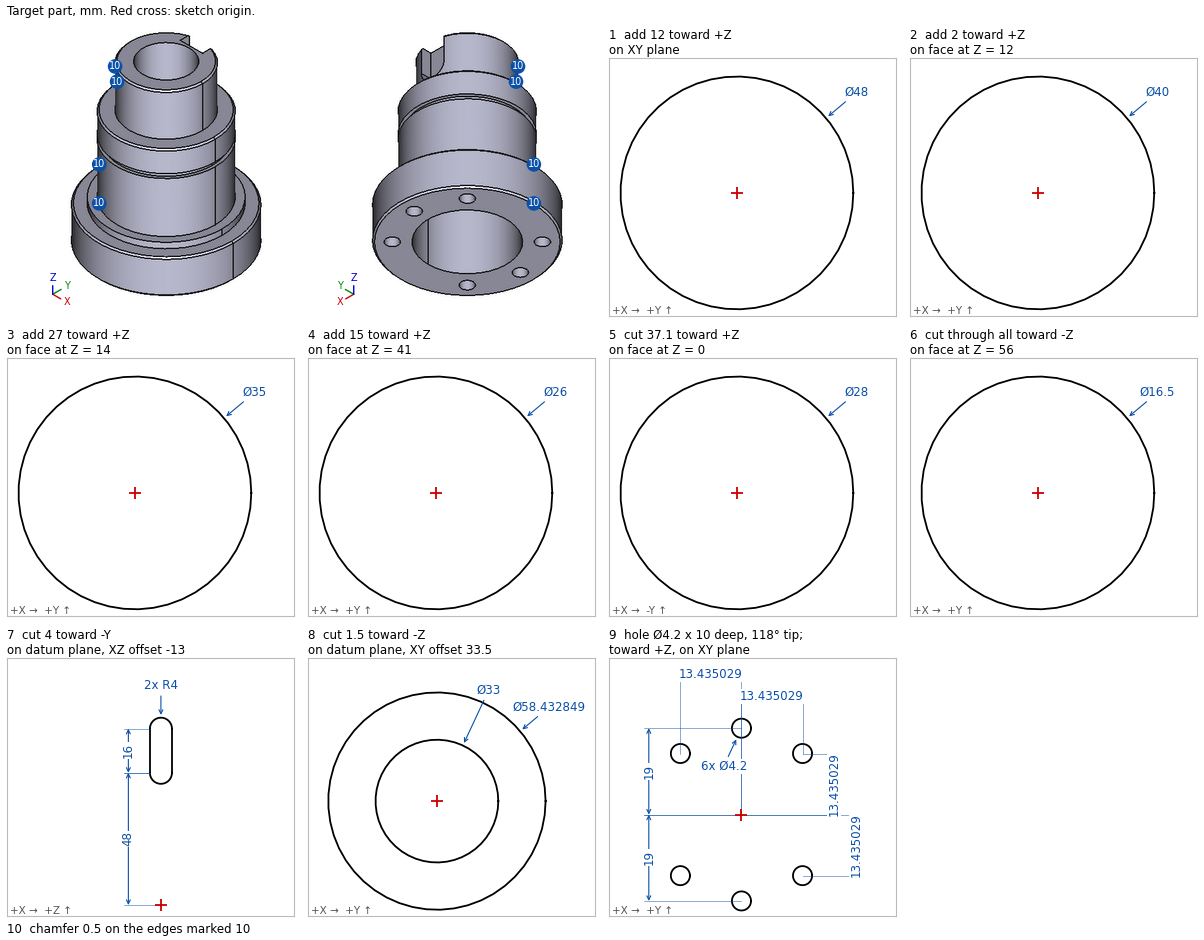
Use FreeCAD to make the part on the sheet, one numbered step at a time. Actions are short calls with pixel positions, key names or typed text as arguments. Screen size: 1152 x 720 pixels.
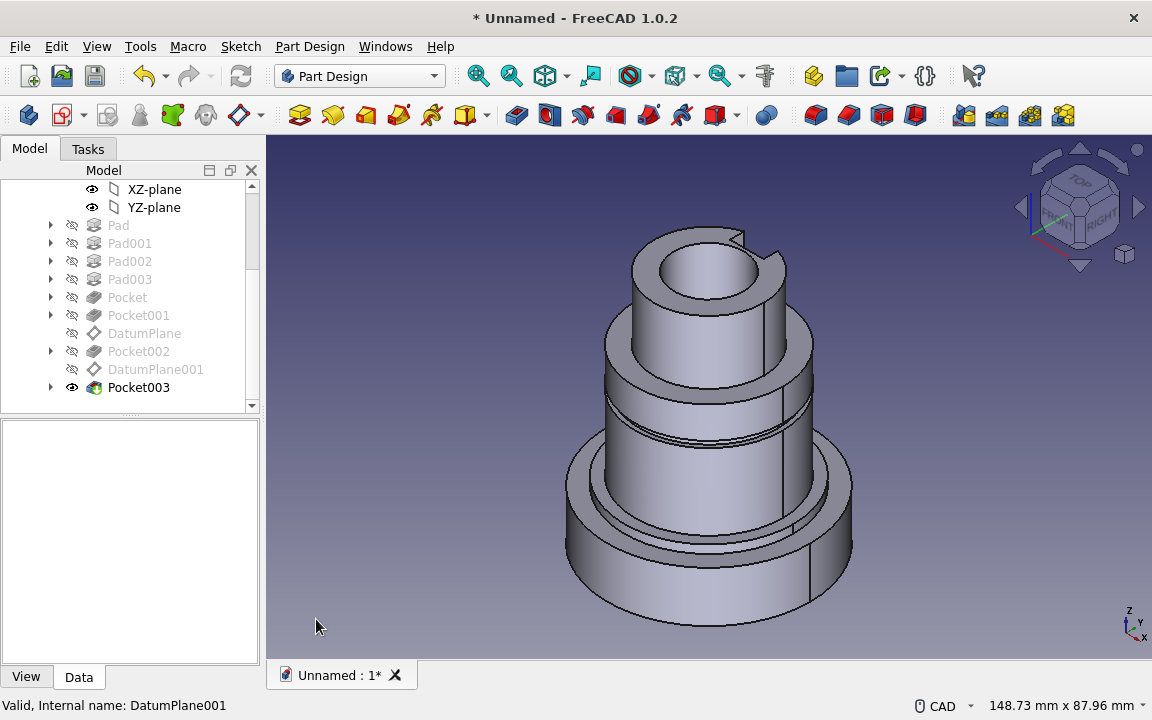
click(62, 116)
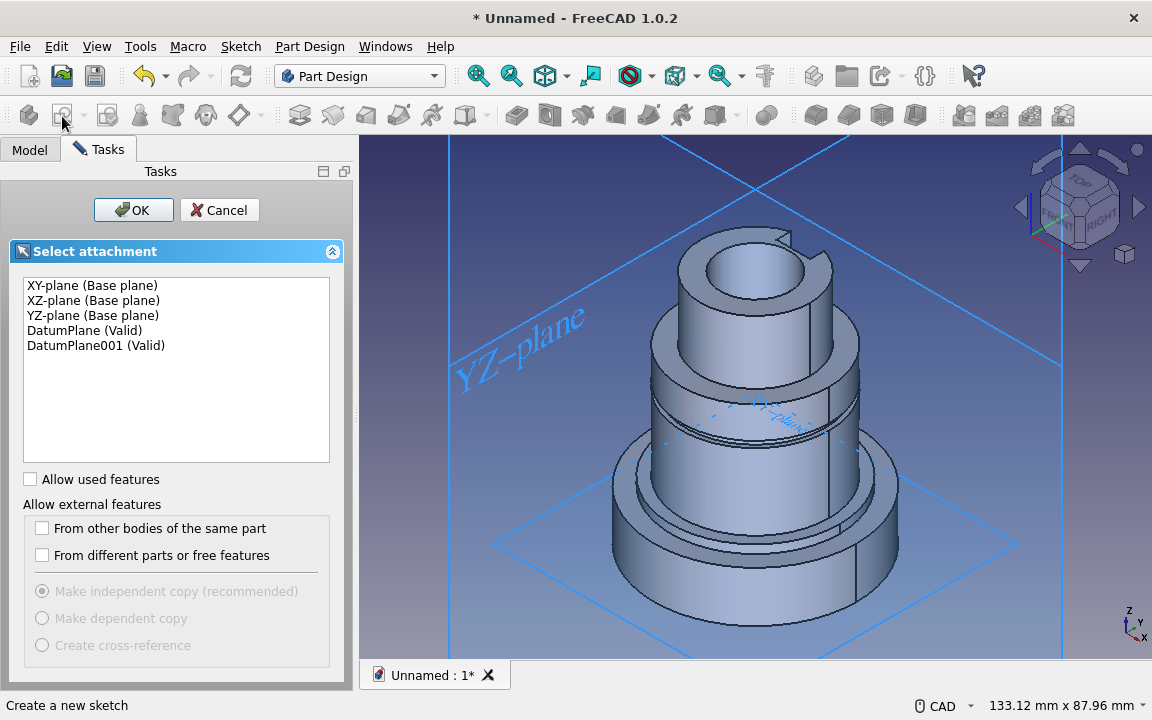
click(84, 286)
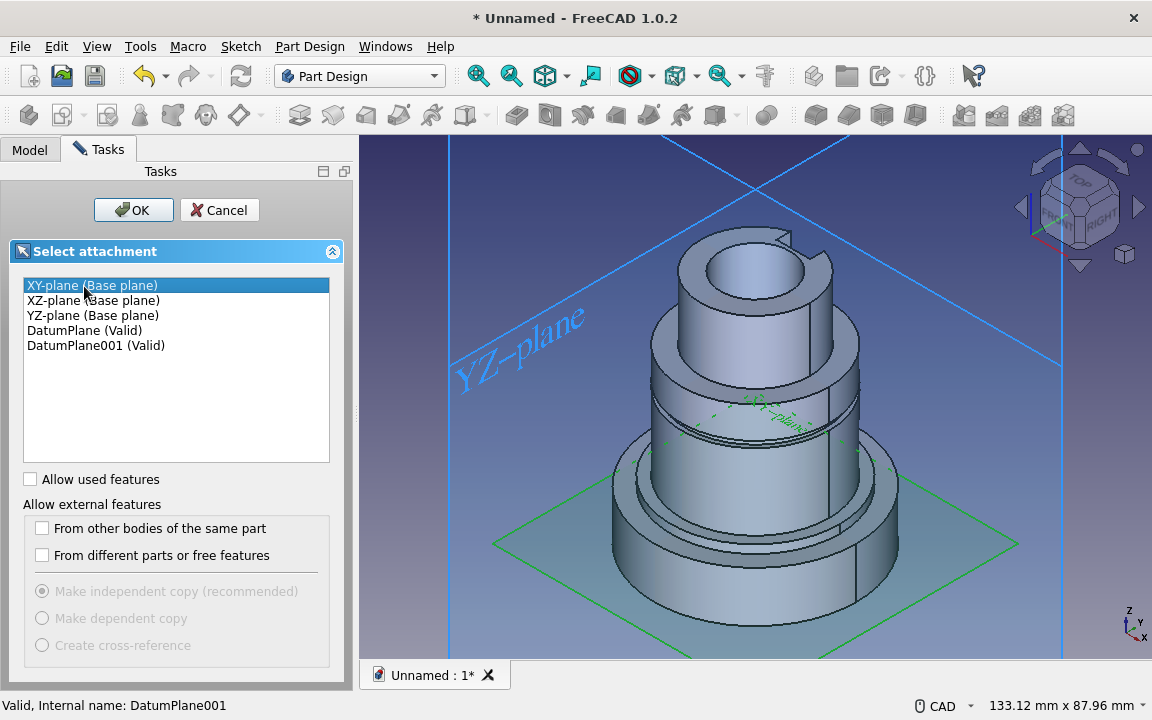
click(134, 210)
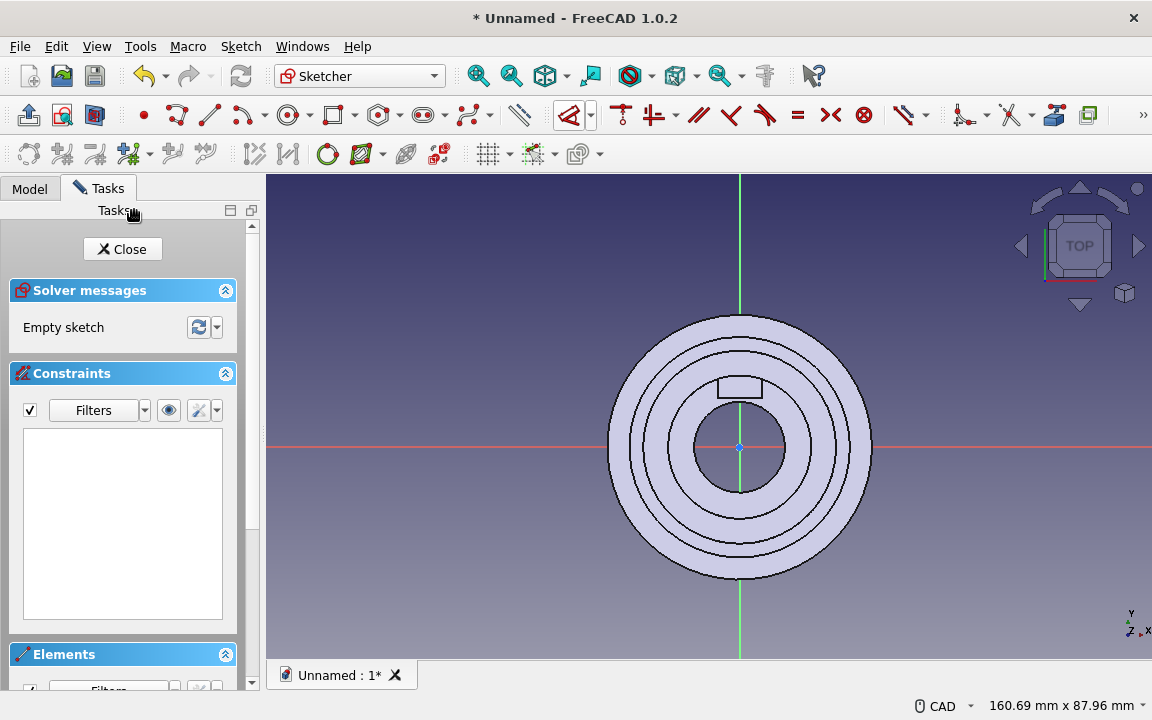
key(q)
key(s)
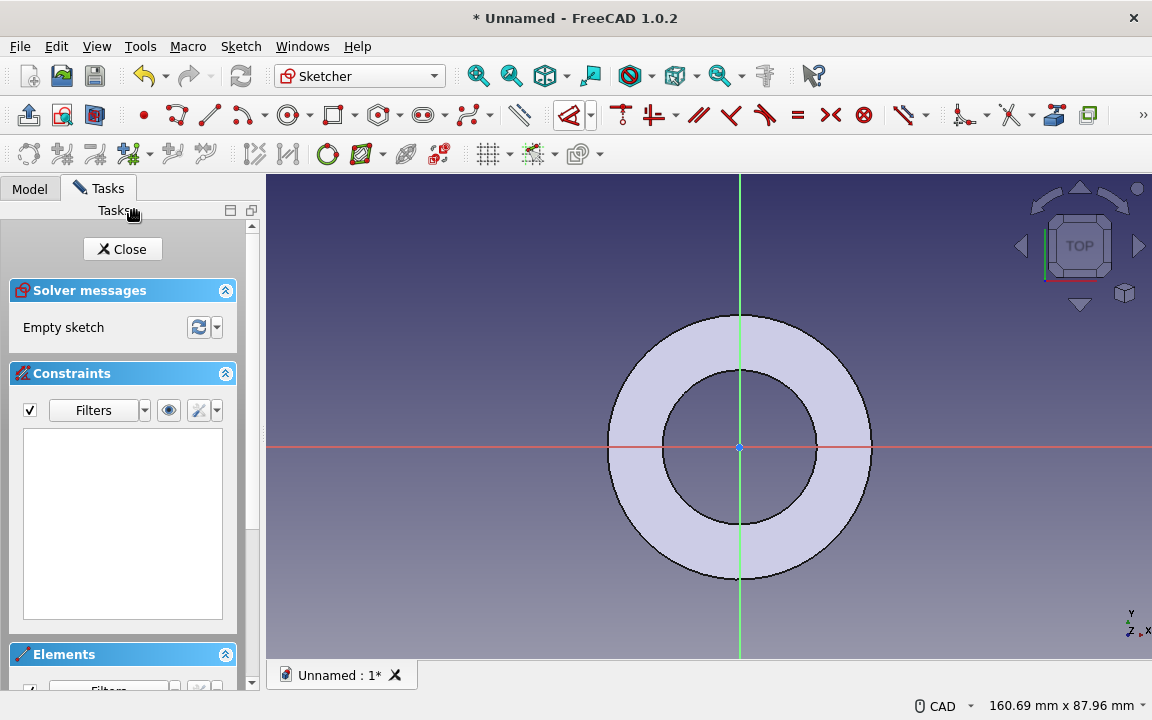
key(g)
key(c)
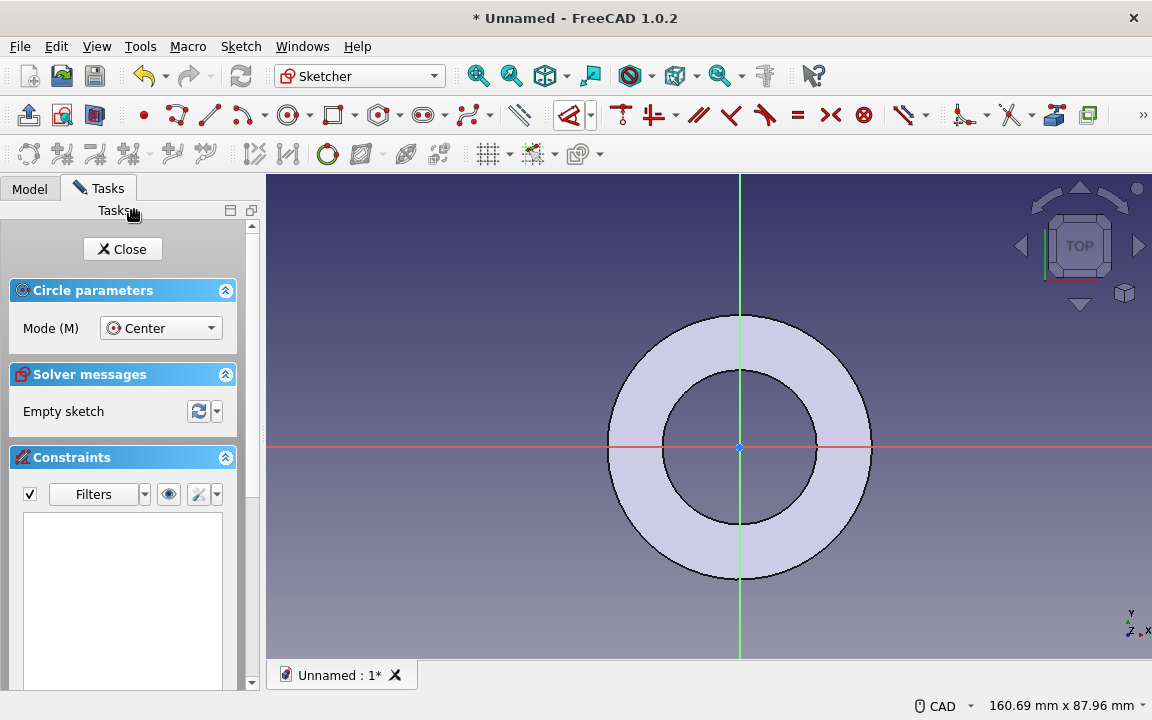
scroll(740, 343, up, 4)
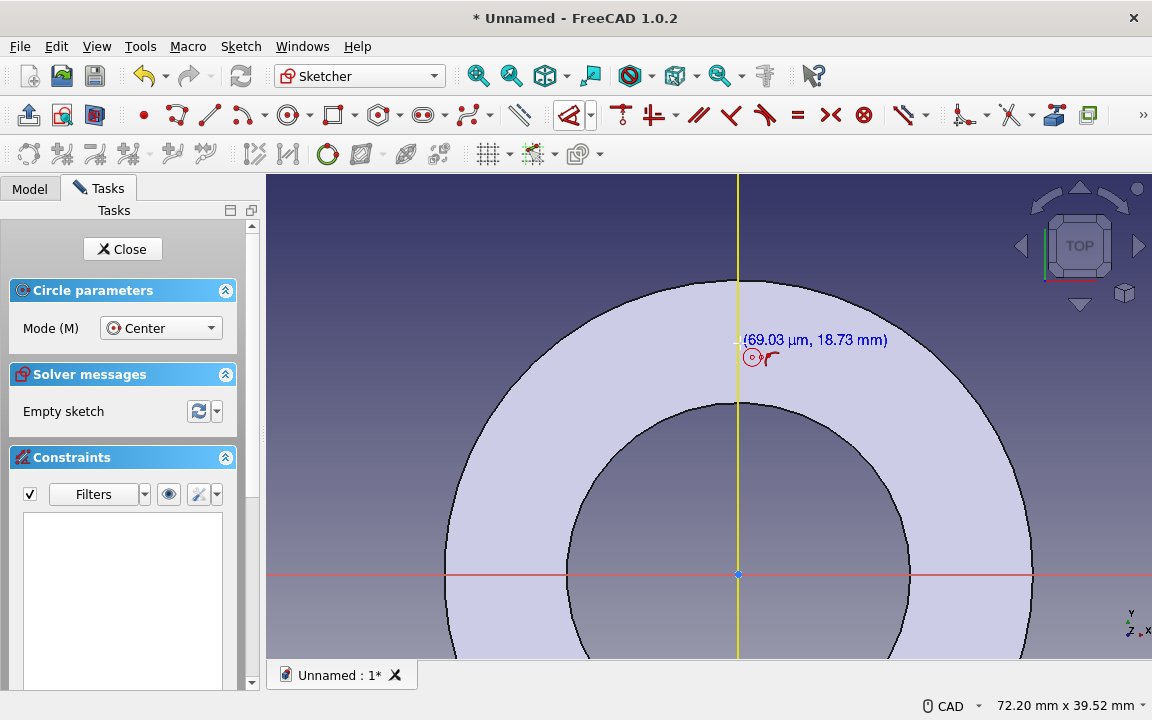
click(738, 341)
click(757, 323)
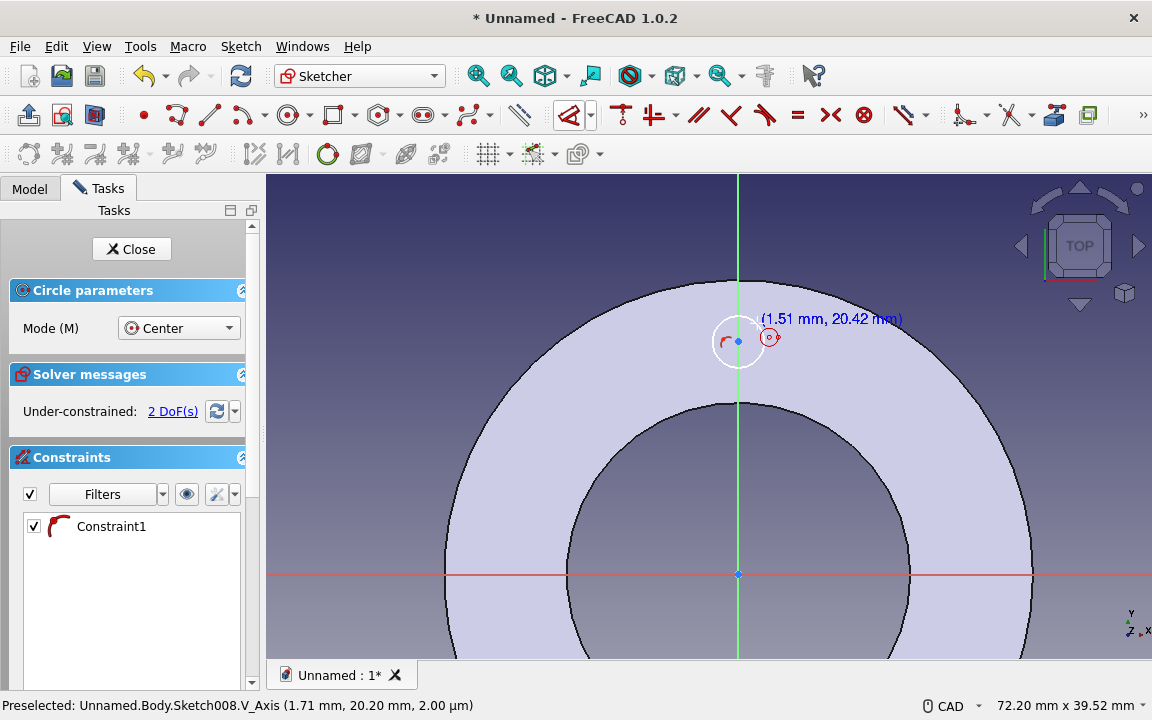
click(903, 410)
click(922, 392)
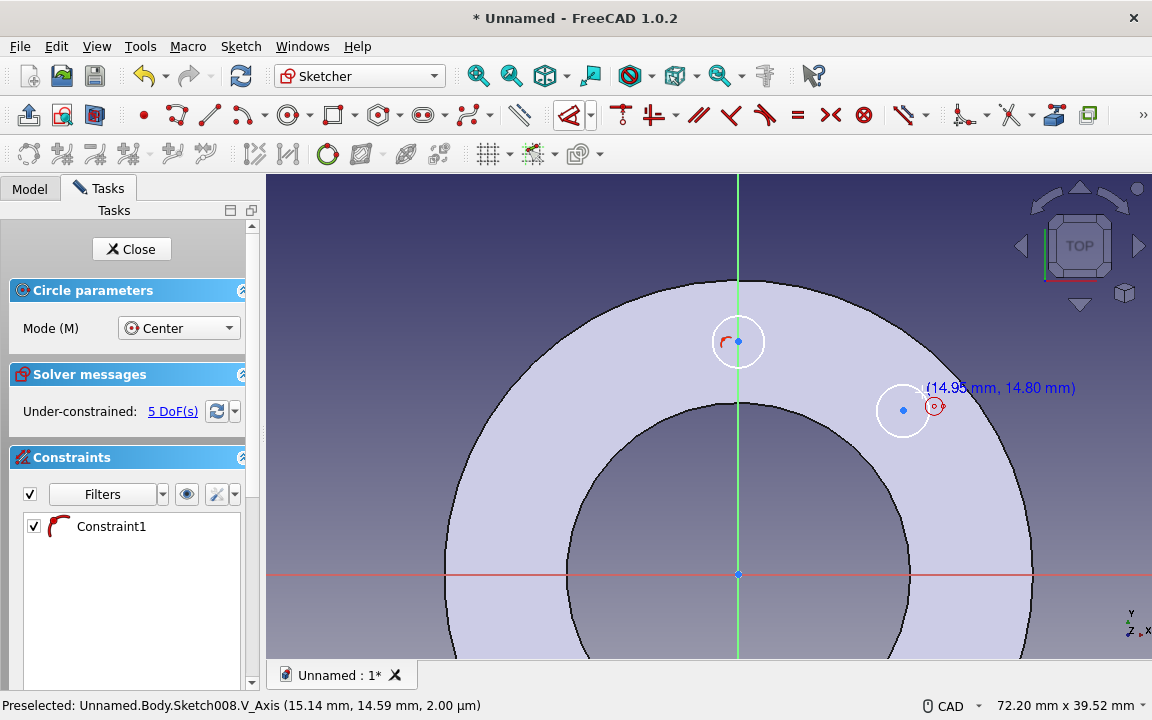
click(574, 410)
click(592, 392)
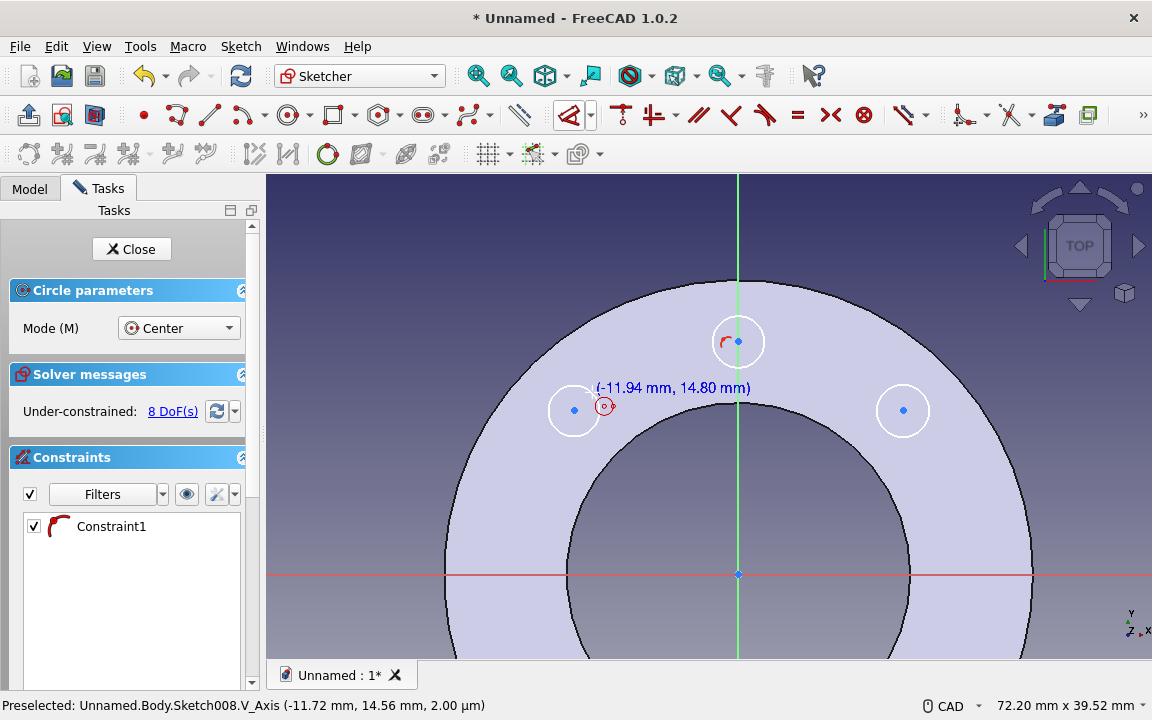
scroll(521, 224, down, 3)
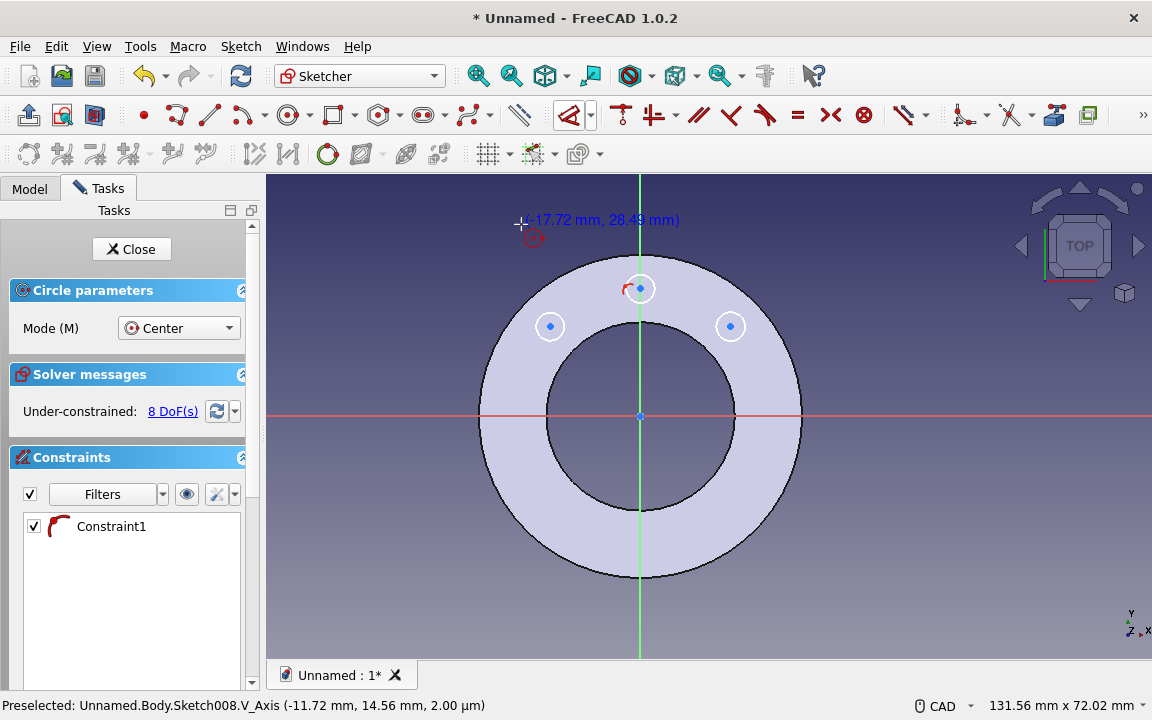
scroll(731, 507, up, 3)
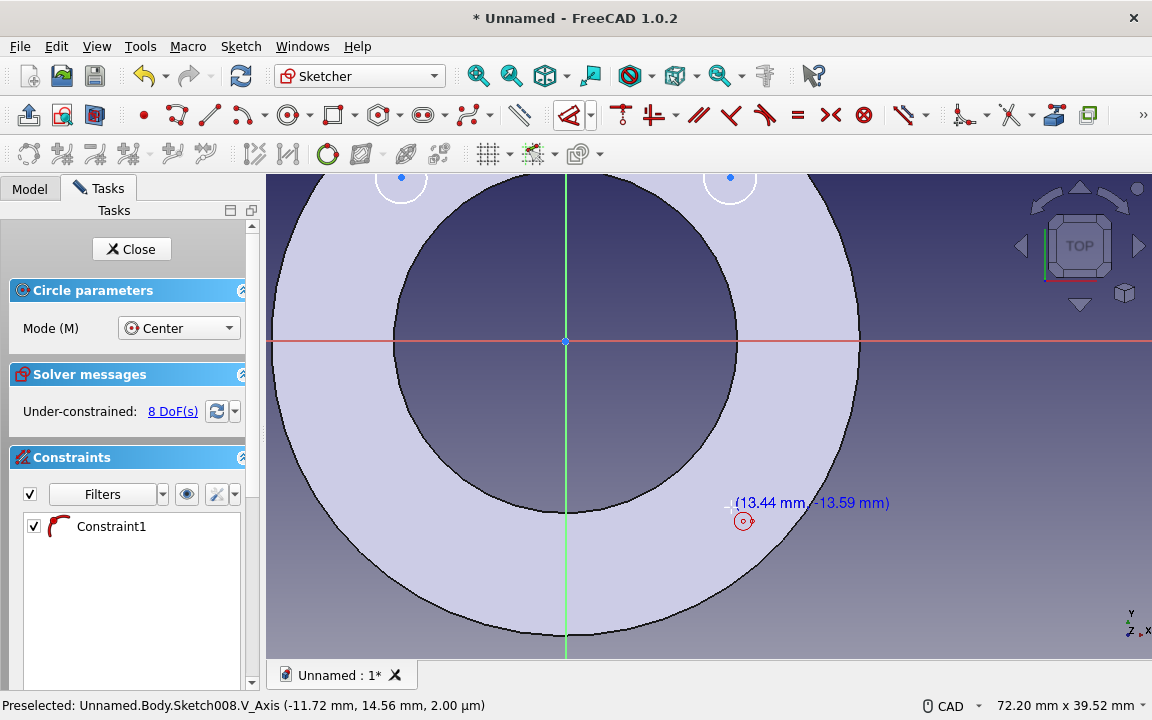
click(731, 506)
click(749, 488)